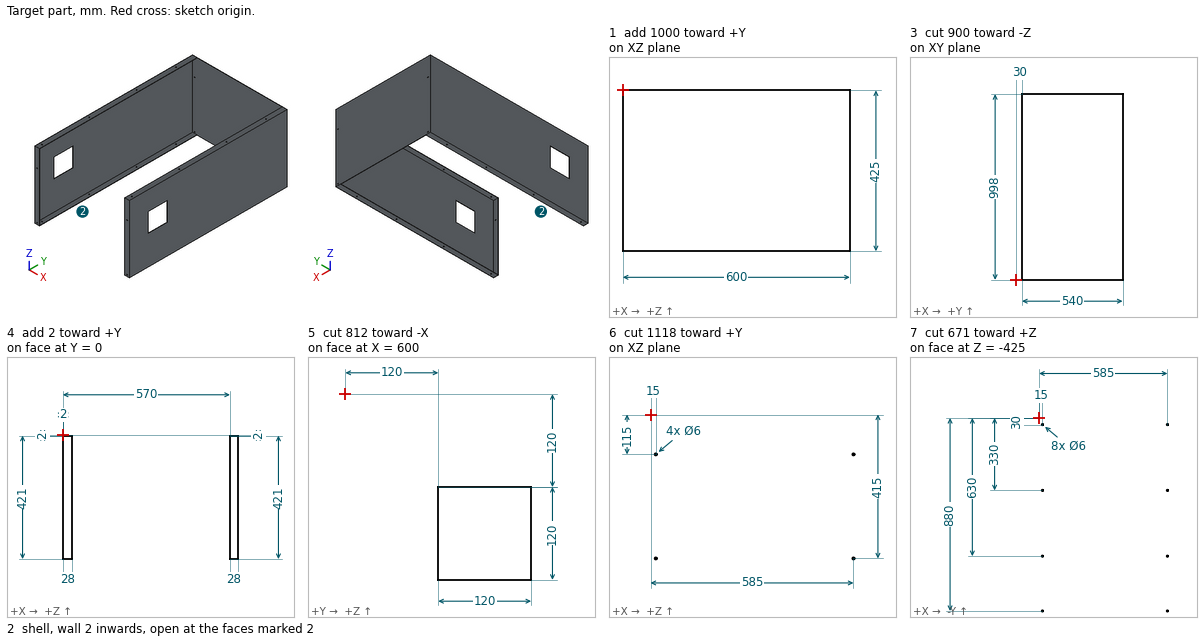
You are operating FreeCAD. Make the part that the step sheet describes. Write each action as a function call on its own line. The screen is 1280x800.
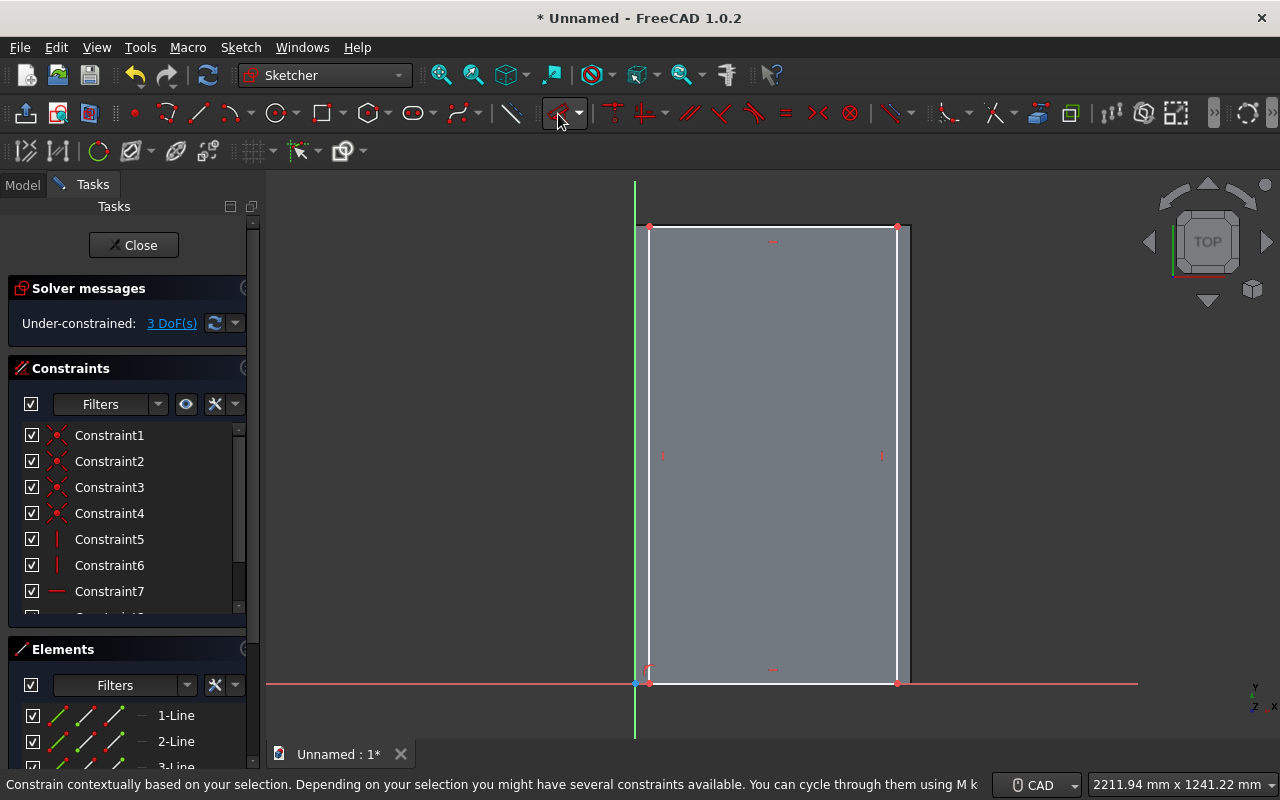
click(649, 364)
click(615, 455)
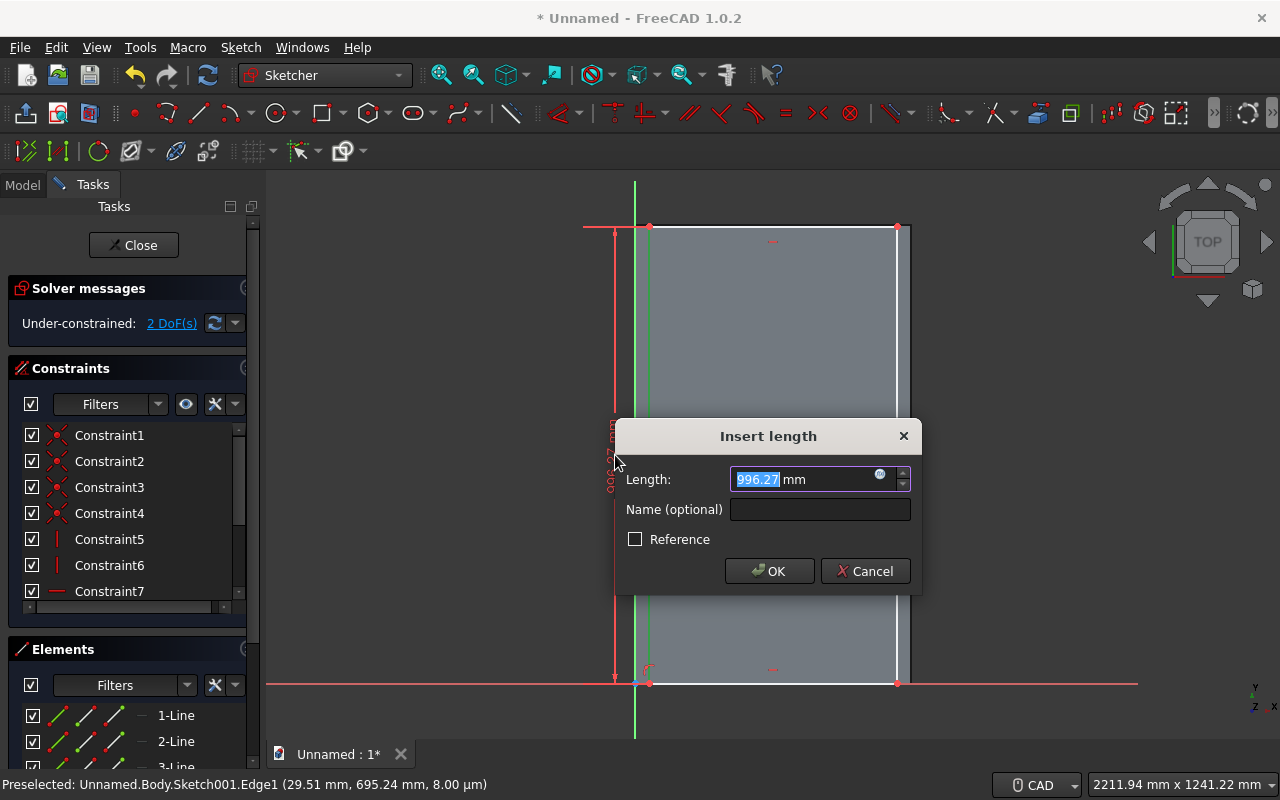
text(998)
key(Return)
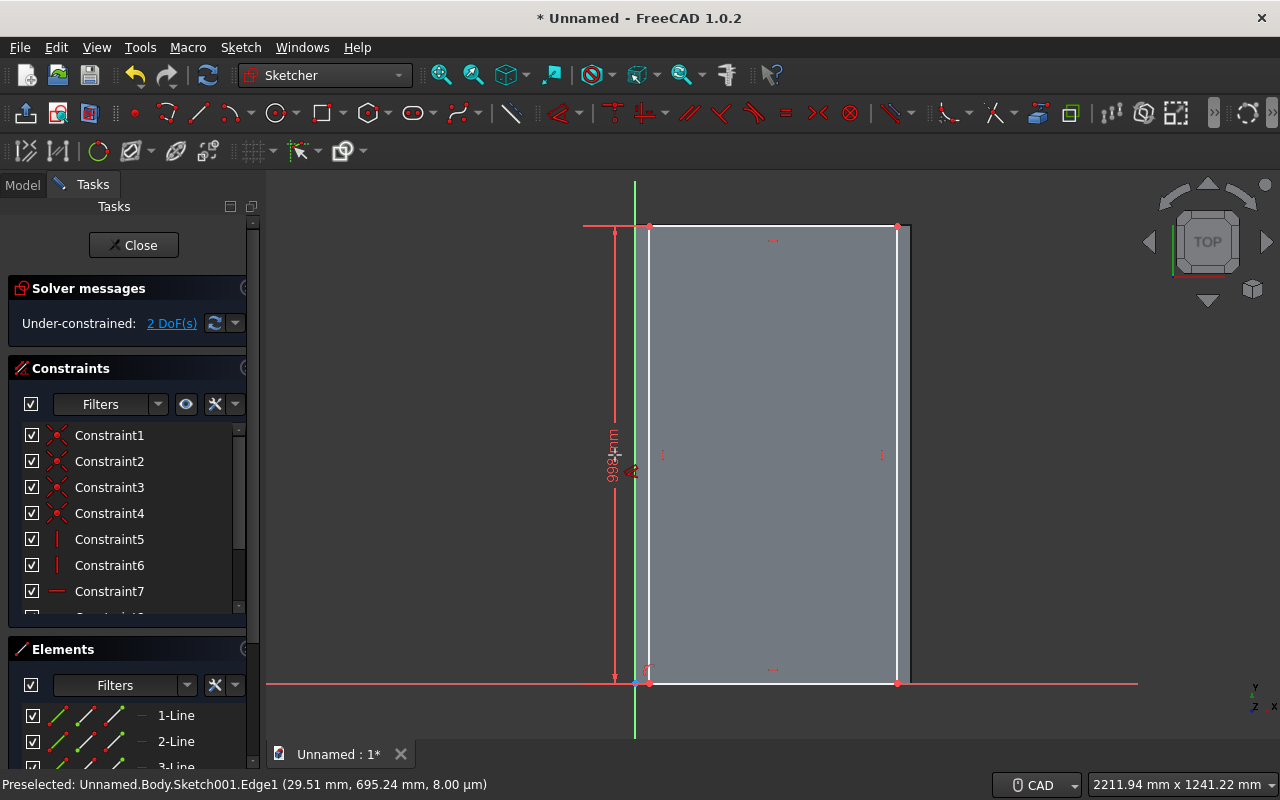
click(723, 684)
click(773, 650)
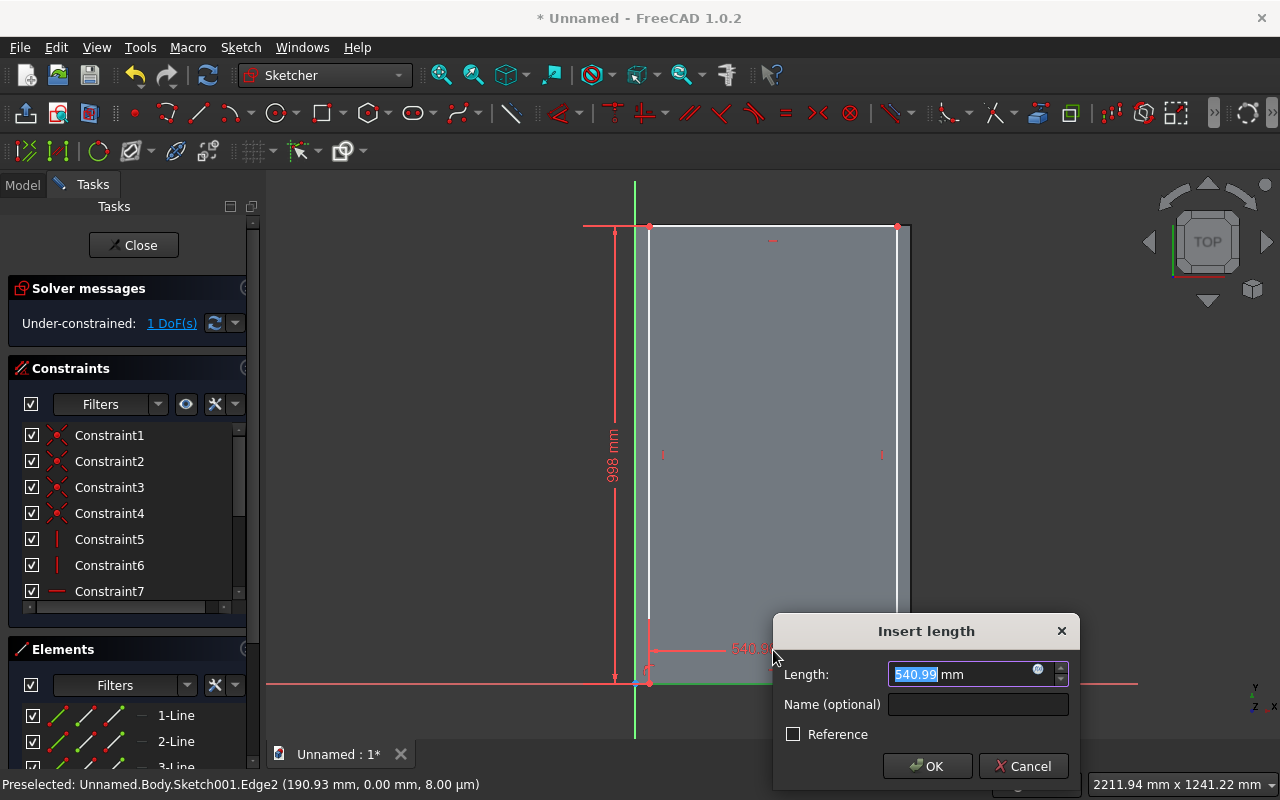
text(540)
key(Return)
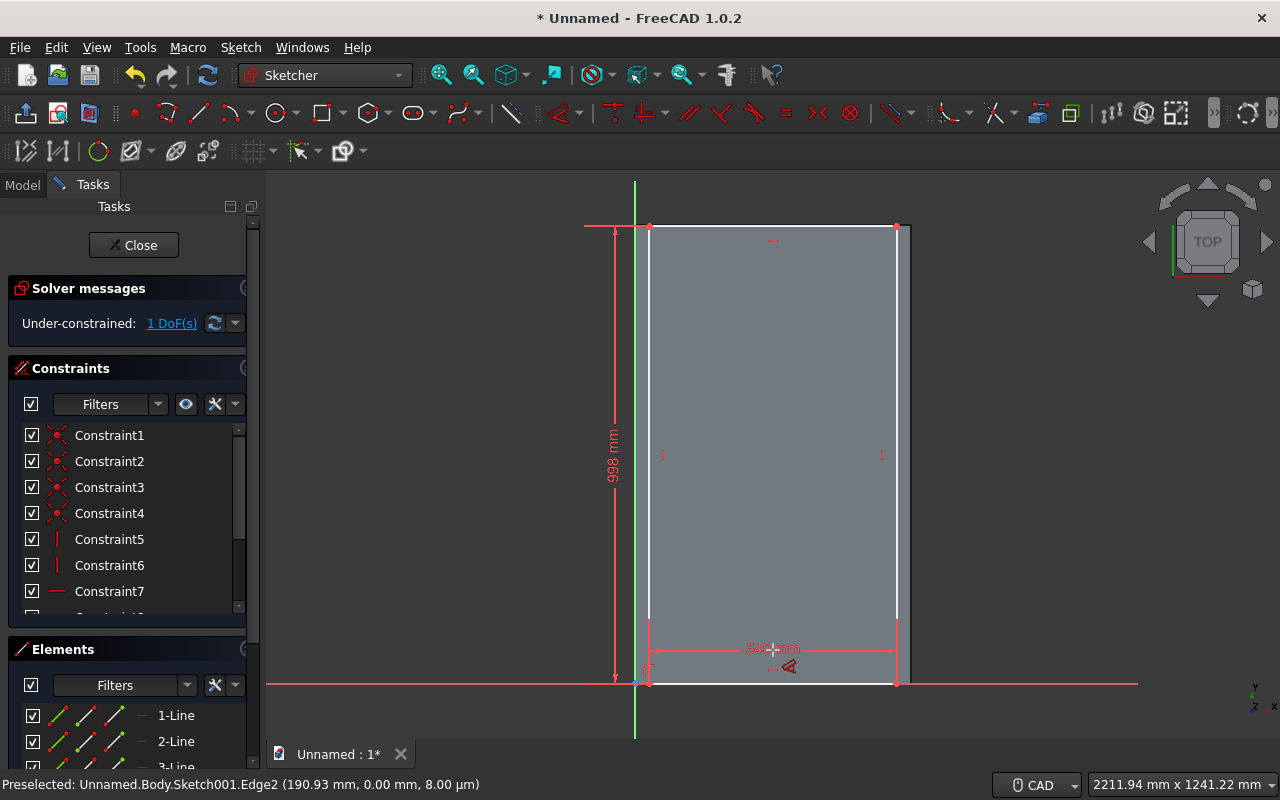
scroll(649, 226, up, 6)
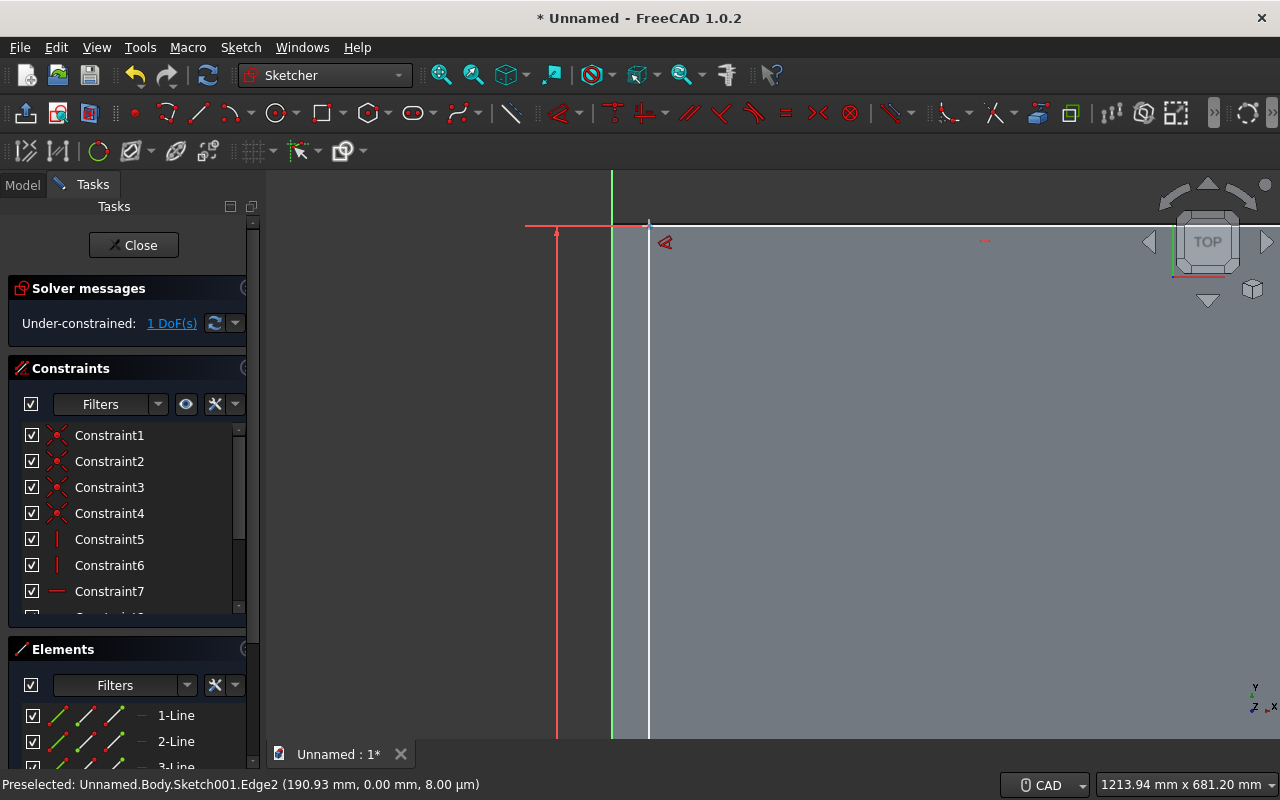
click(649, 226)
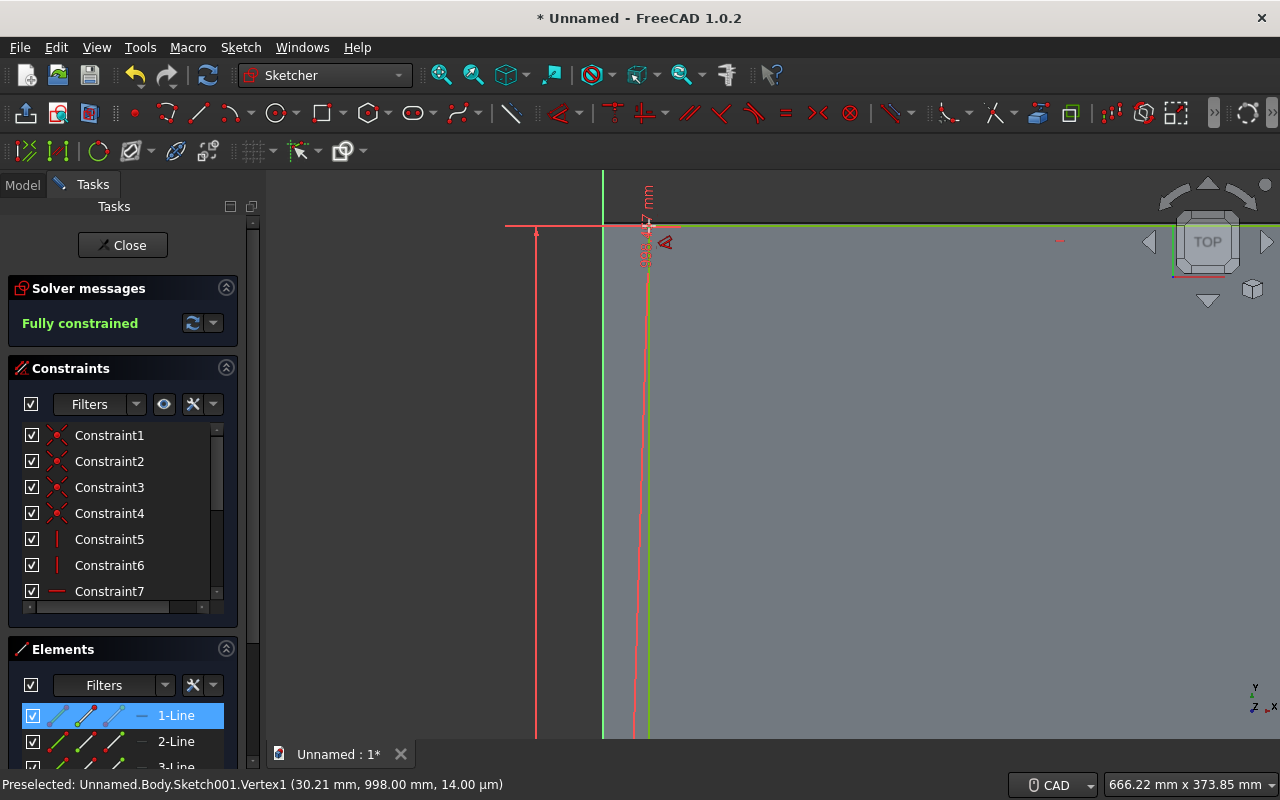
key(Escape)
key(Escape)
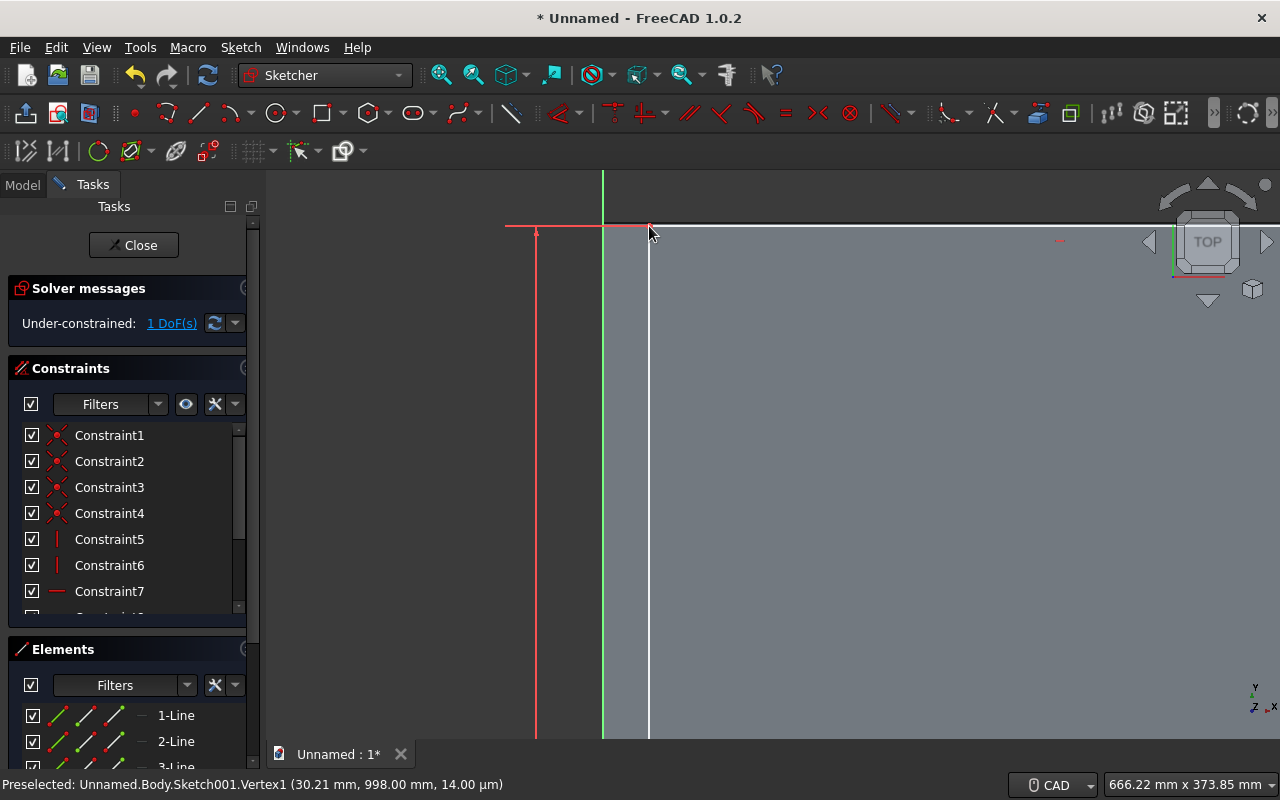
click(649, 226)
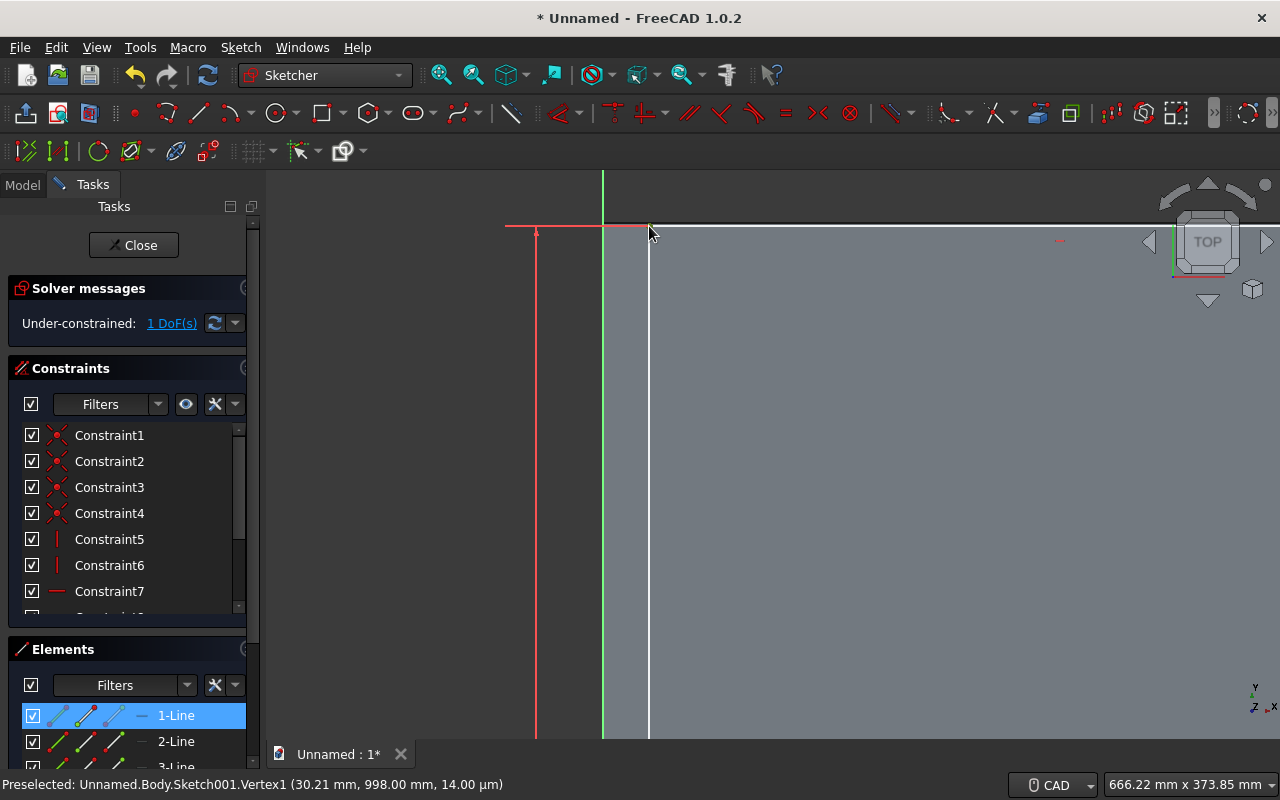
key(l)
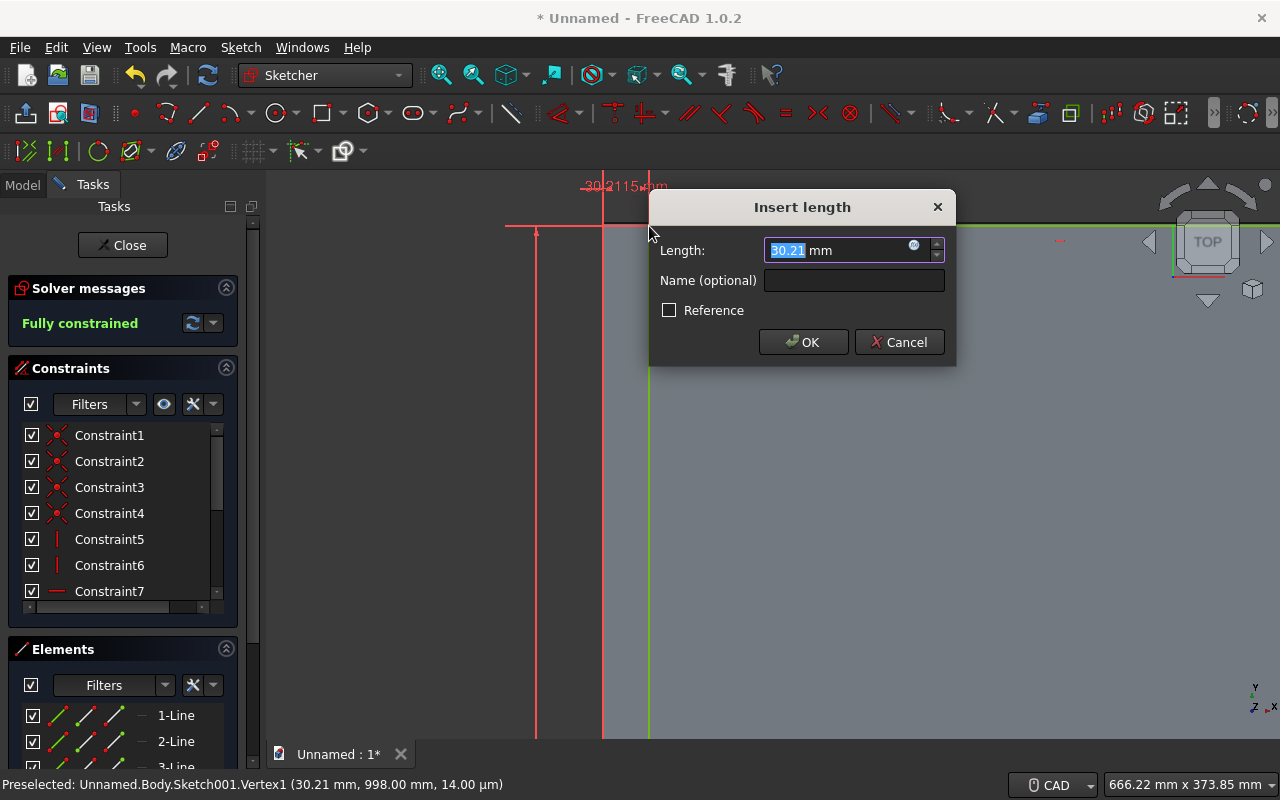
text(30)
key(Return)